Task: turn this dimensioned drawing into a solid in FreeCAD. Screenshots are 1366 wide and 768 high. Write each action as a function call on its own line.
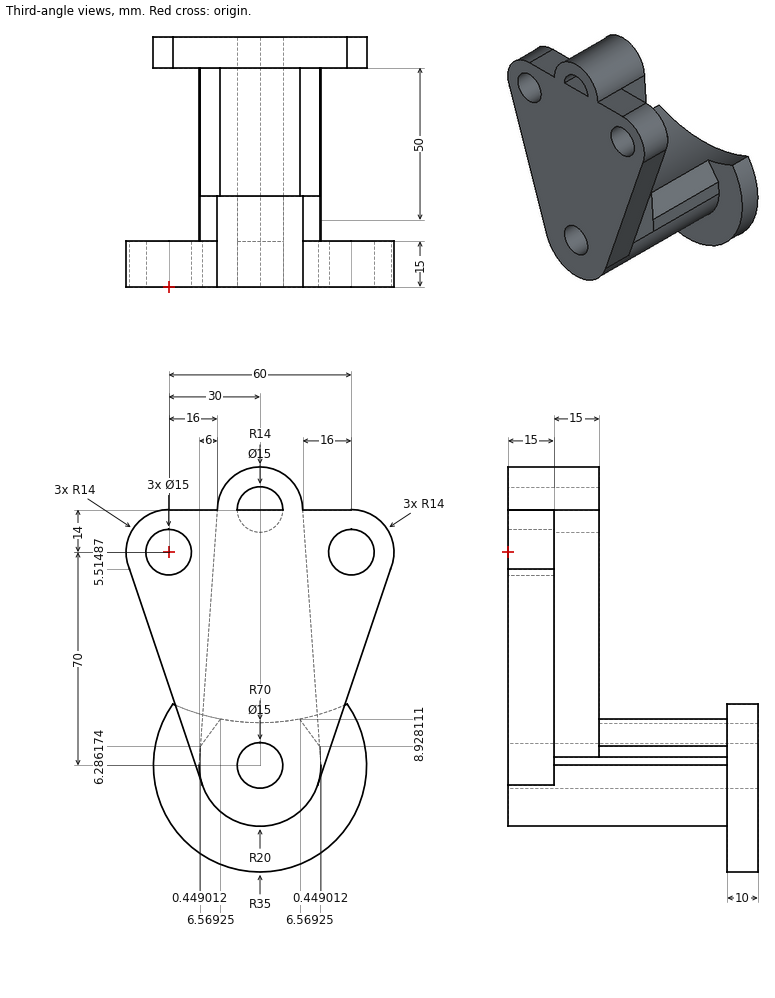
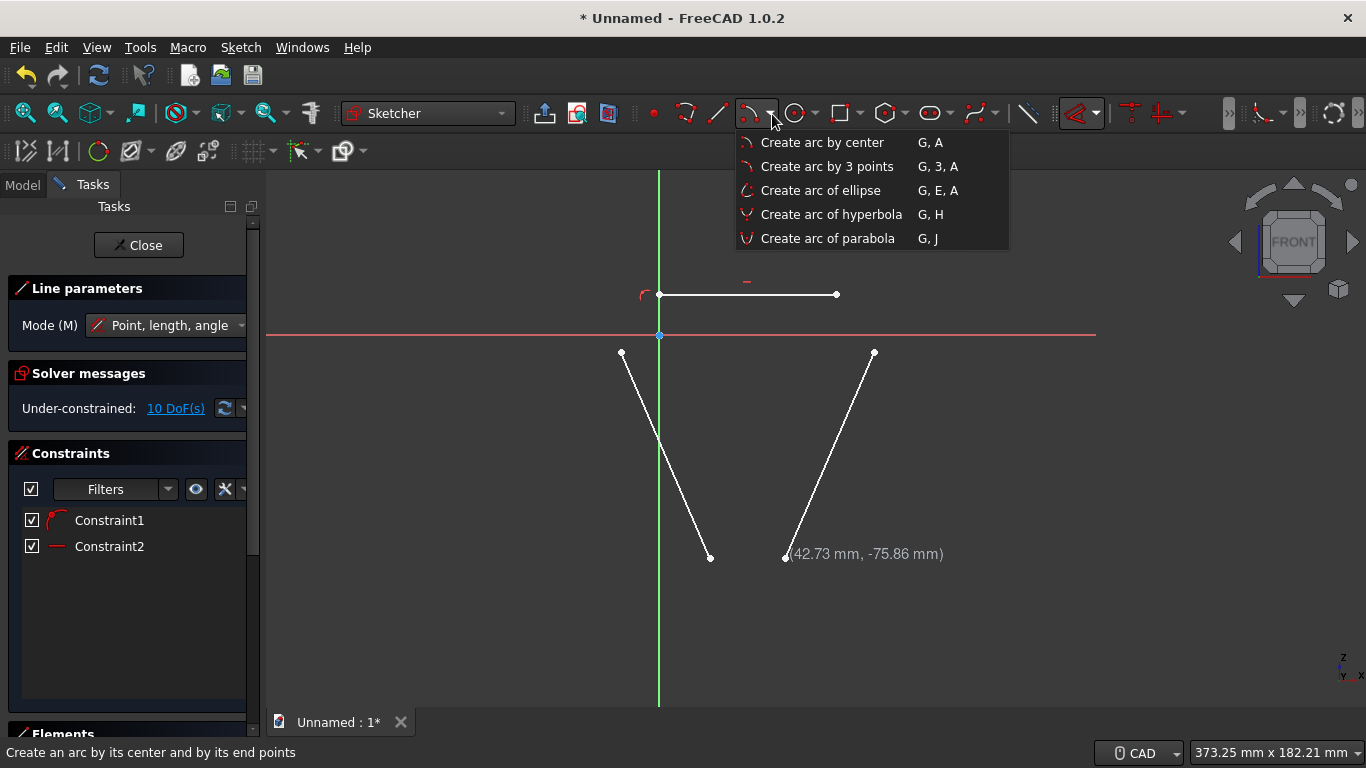
click(872, 166)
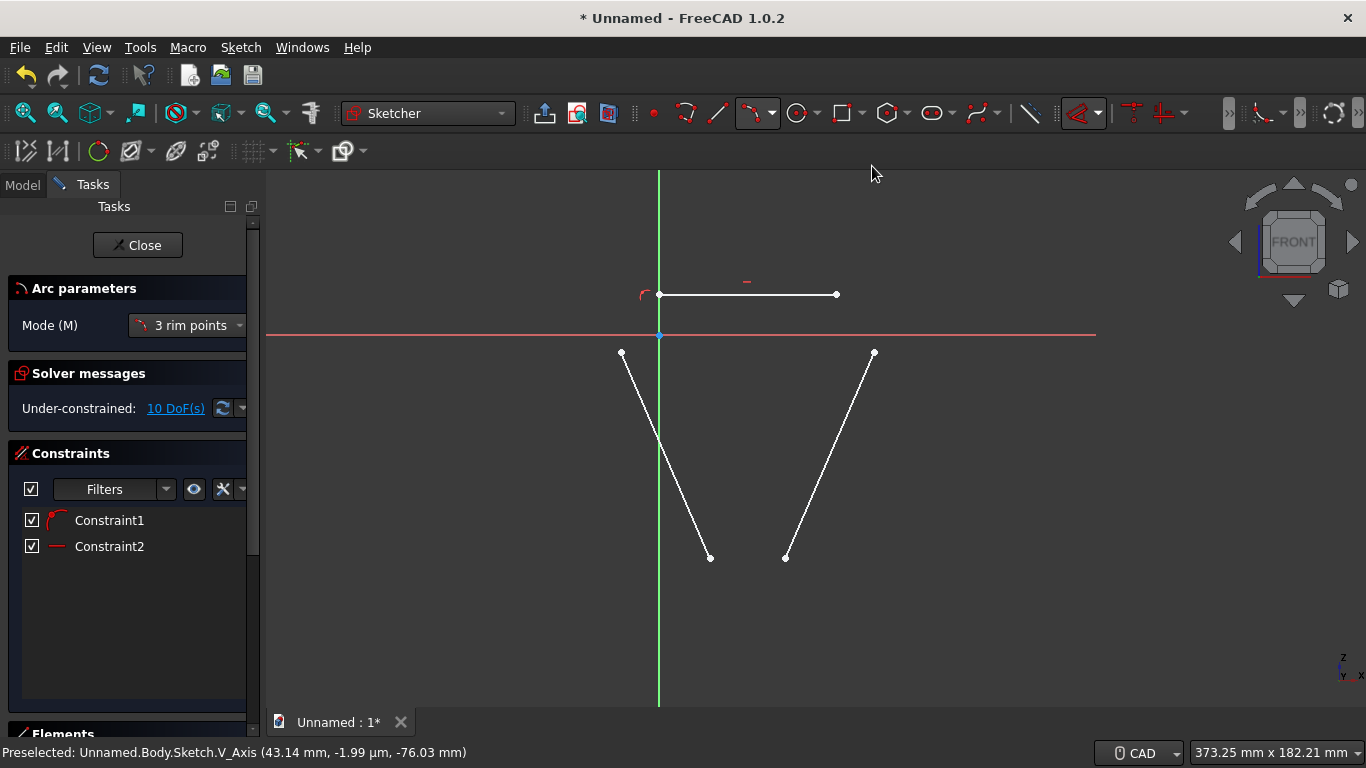
click(621, 353)
click(659, 295)
click(625, 313)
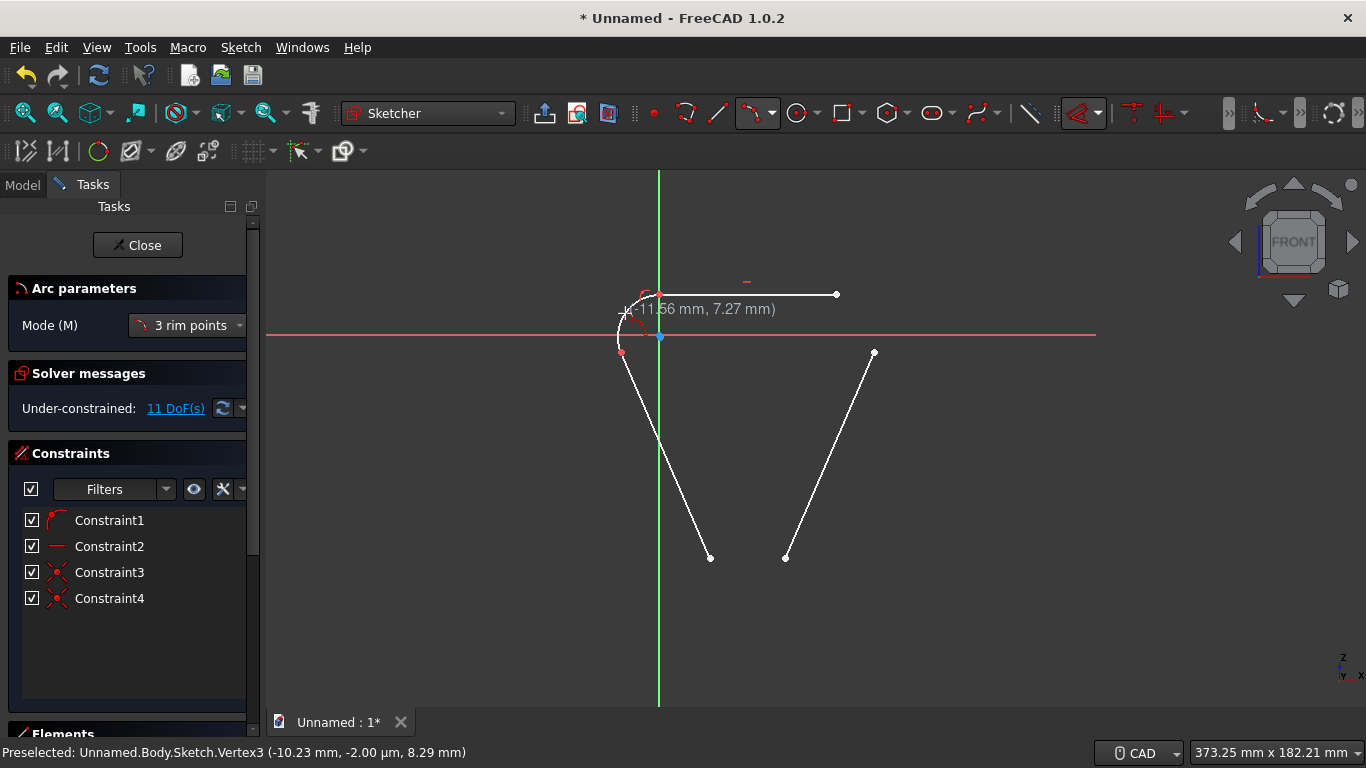
click(836, 295)
click(874, 353)
click(870, 313)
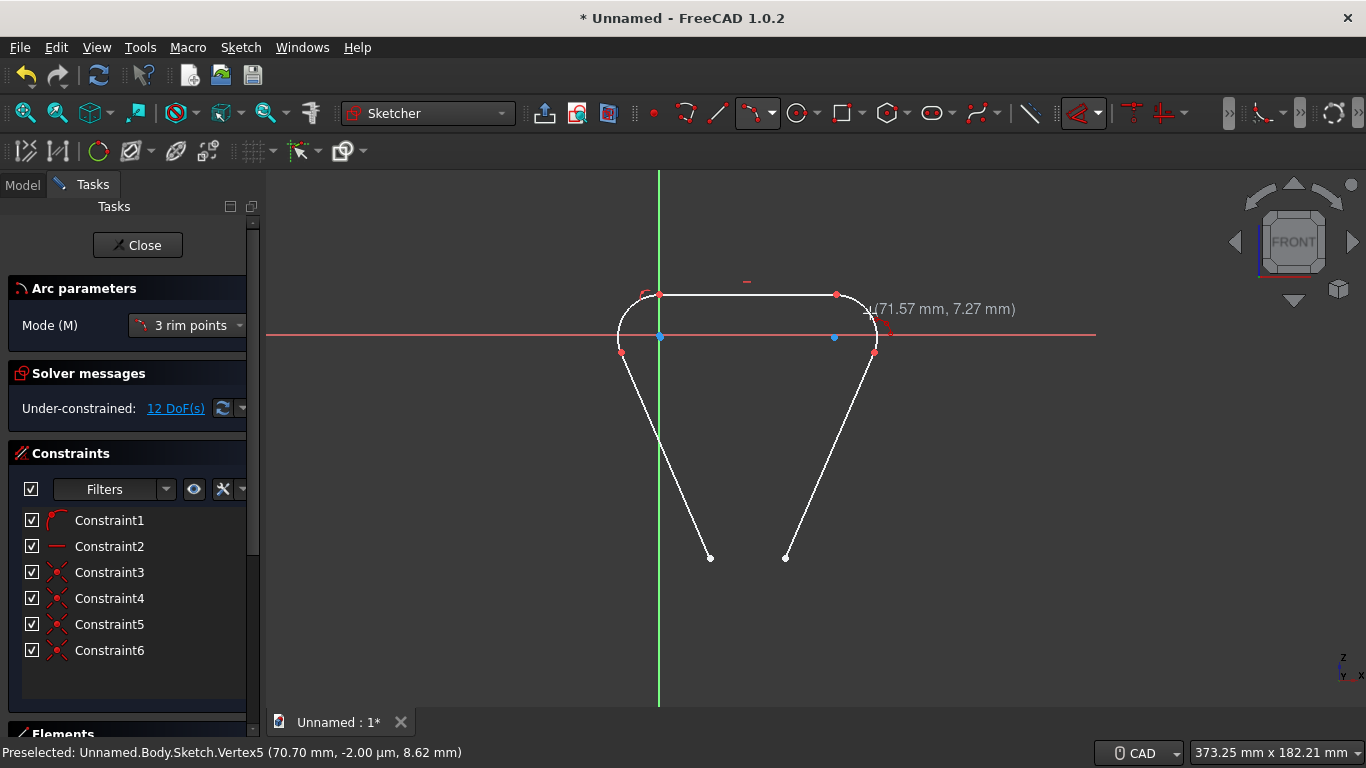
click(785, 559)
click(710, 559)
click(747, 583)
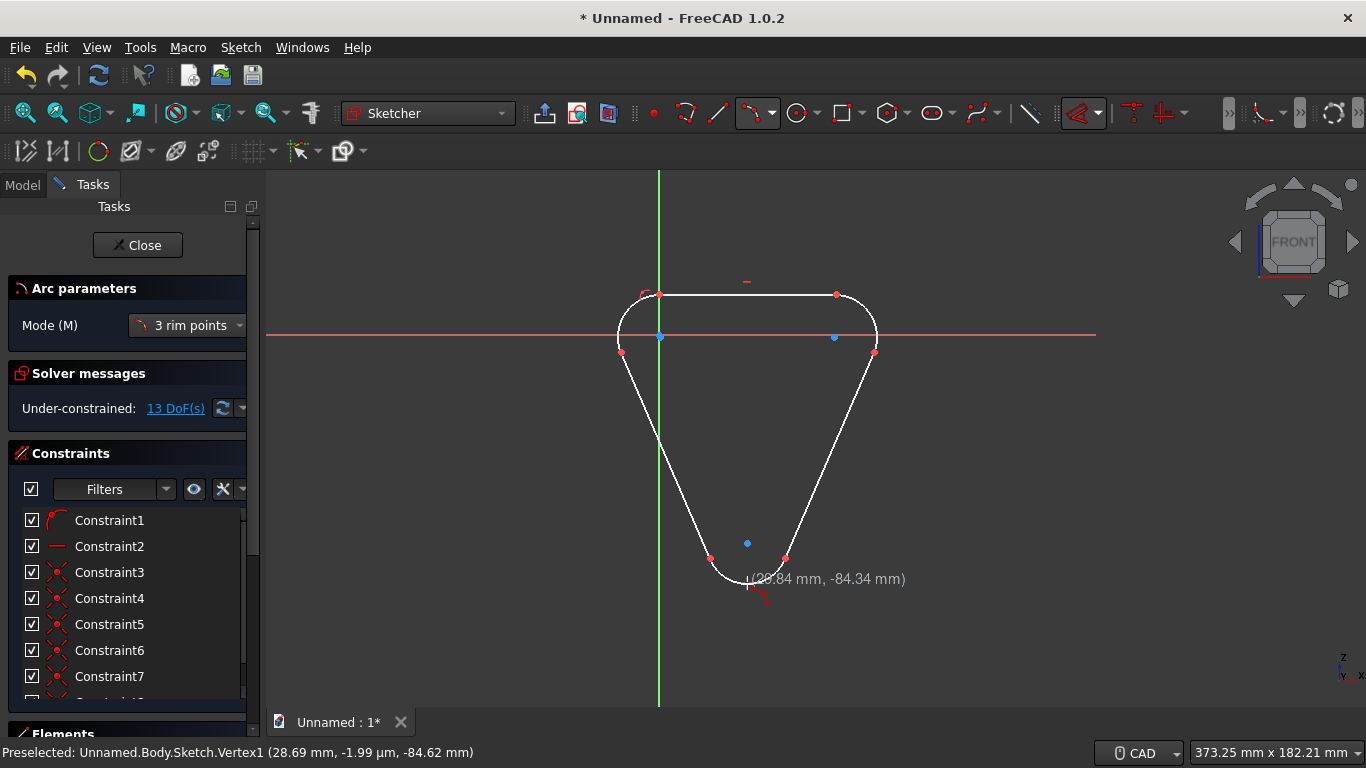
click(798, 114)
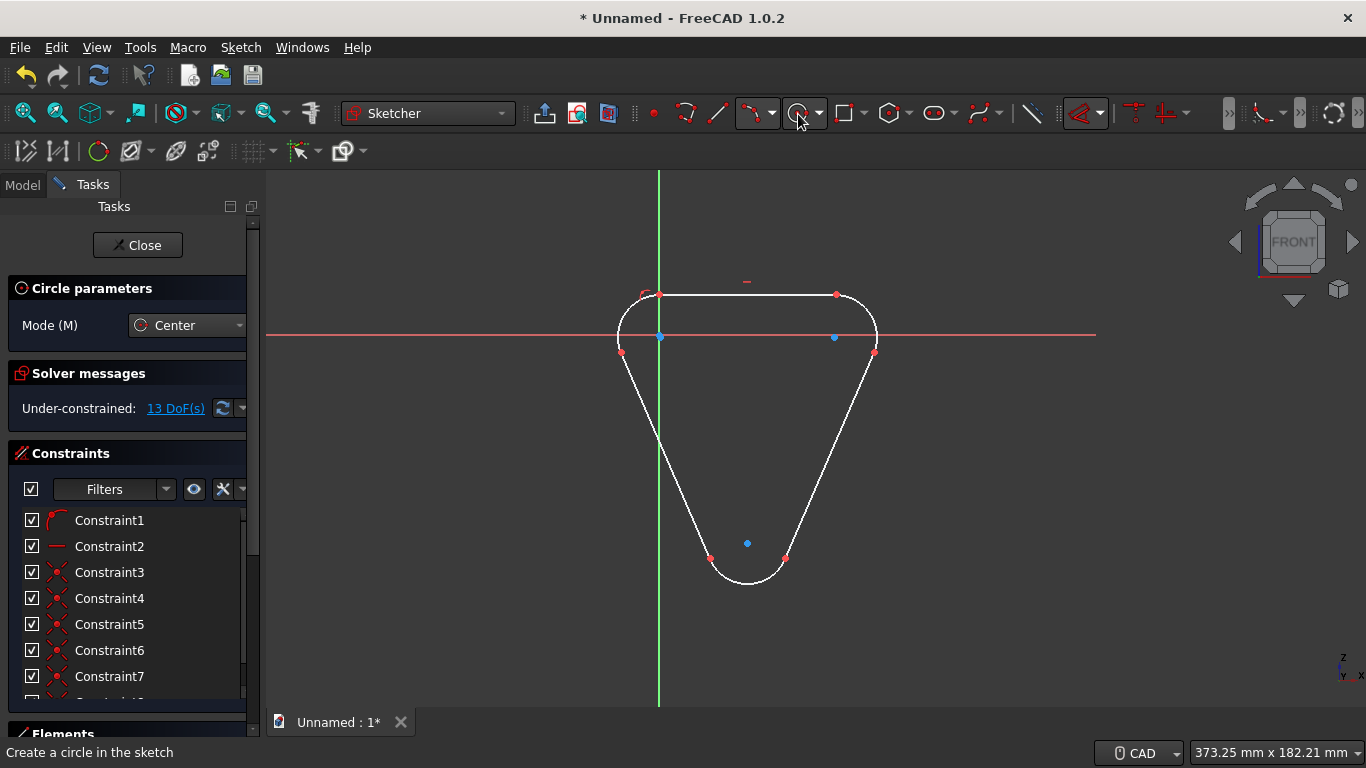
click(659, 335)
move(675, 320)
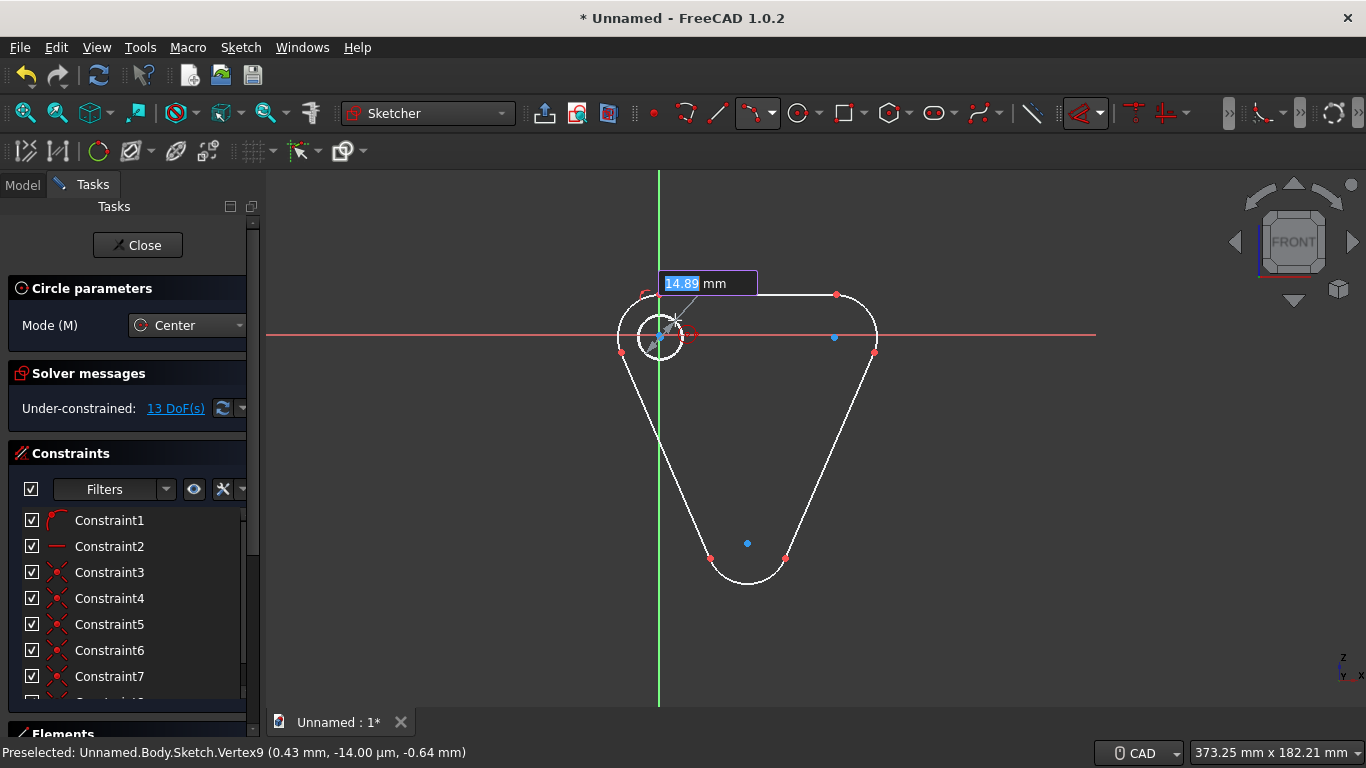
text(15)
key(Return)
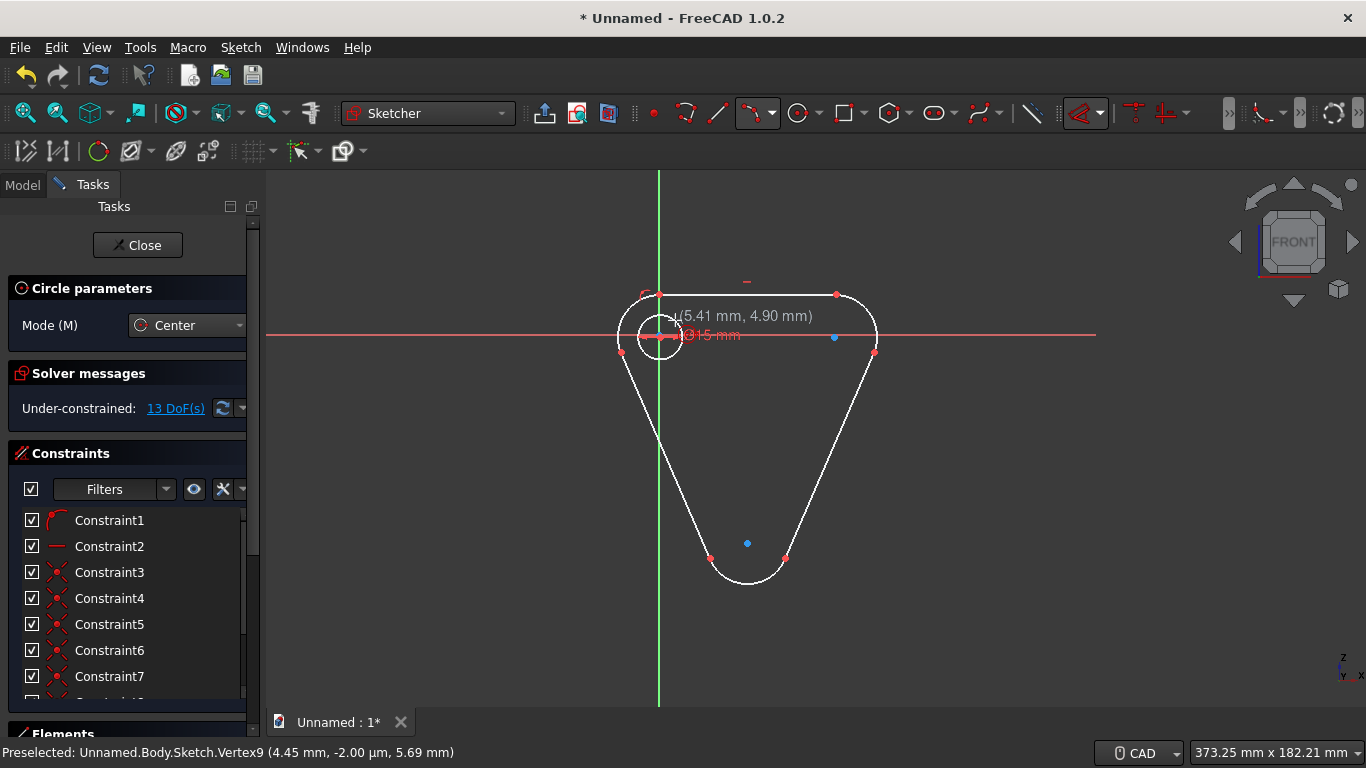
click(836, 335)
move(852, 320)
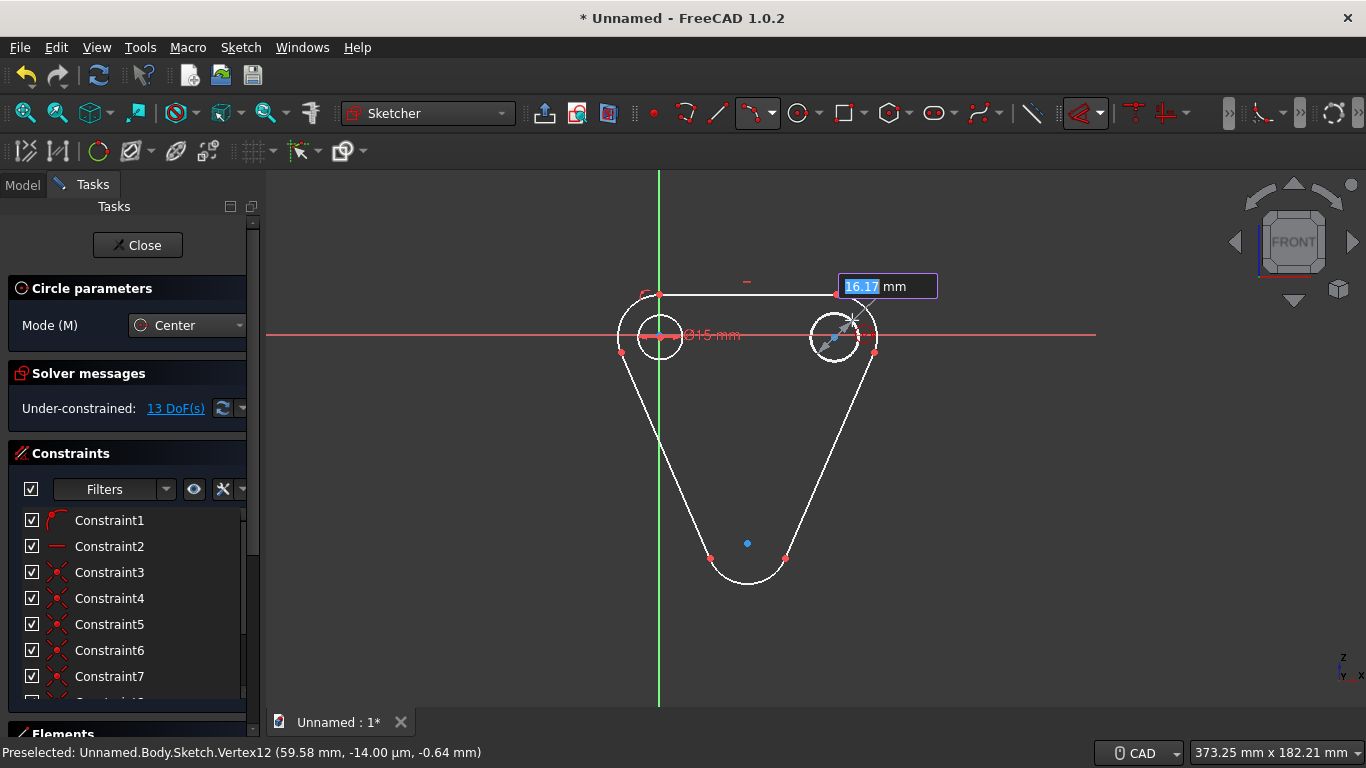
text(15)
key(Return)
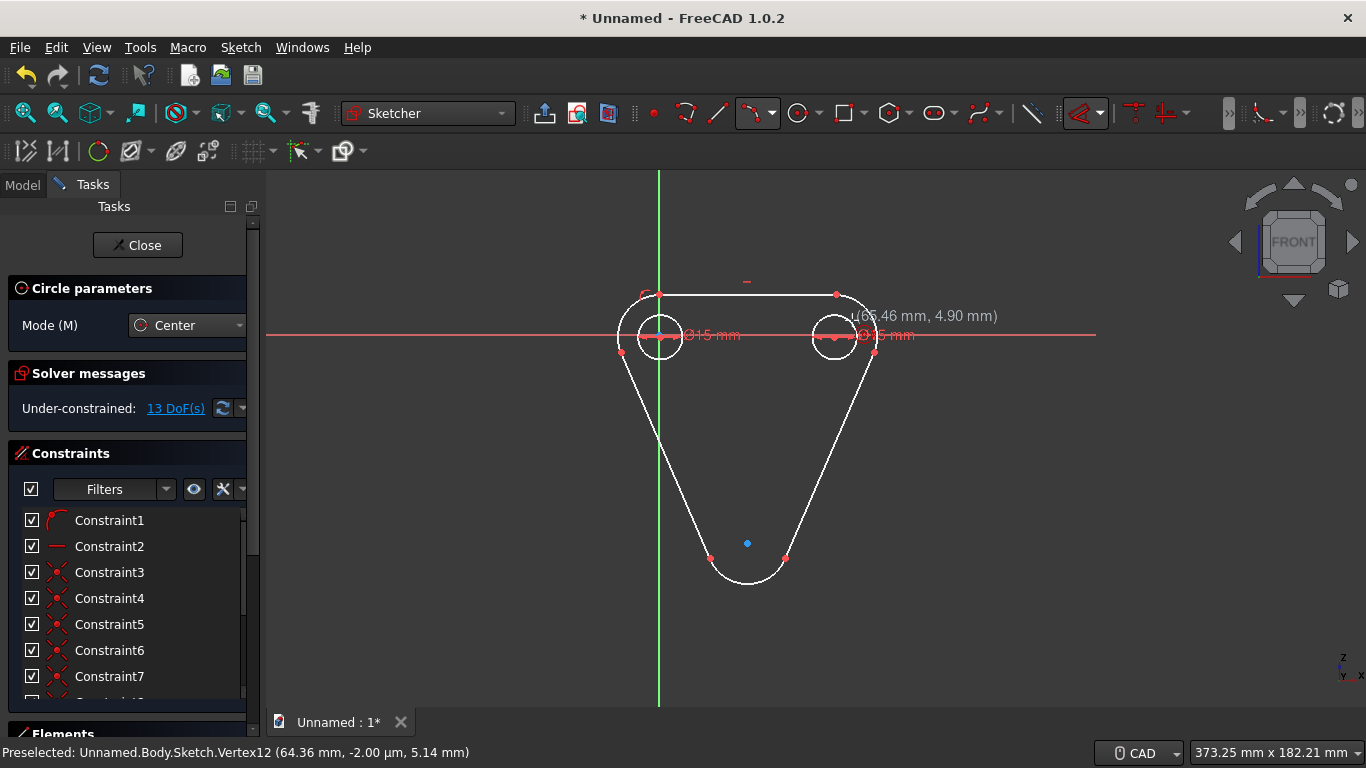
click(747, 542)
move(763, 526)